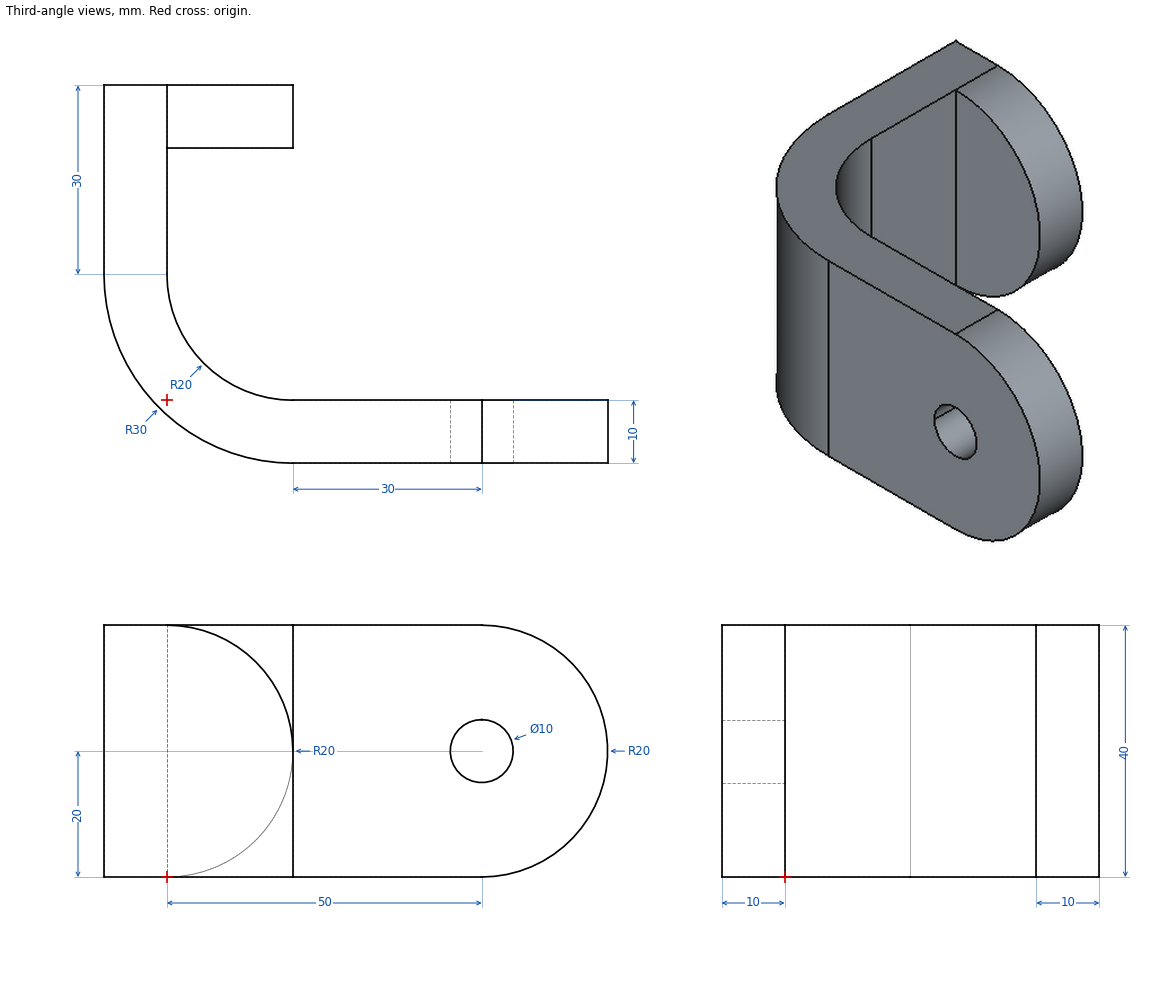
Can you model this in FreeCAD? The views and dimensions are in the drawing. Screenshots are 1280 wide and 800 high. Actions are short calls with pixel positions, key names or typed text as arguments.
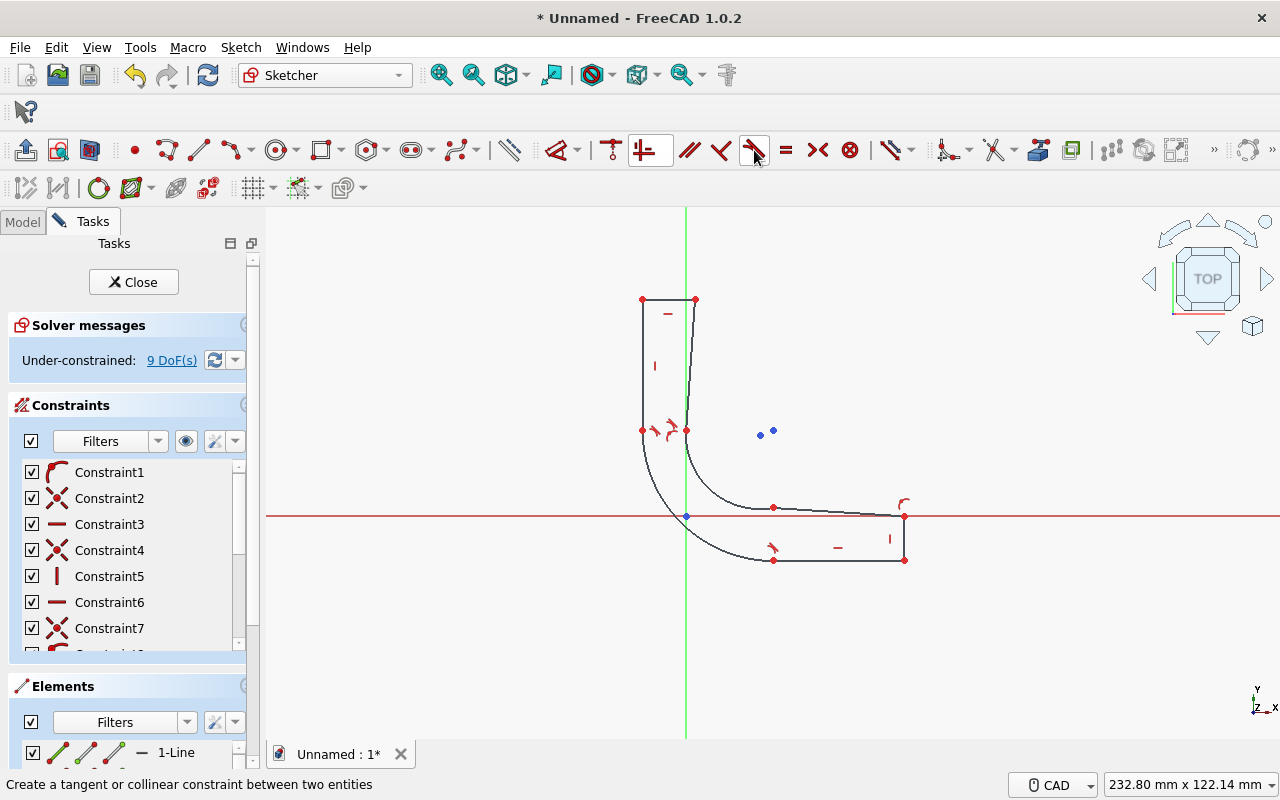
click(865, 514)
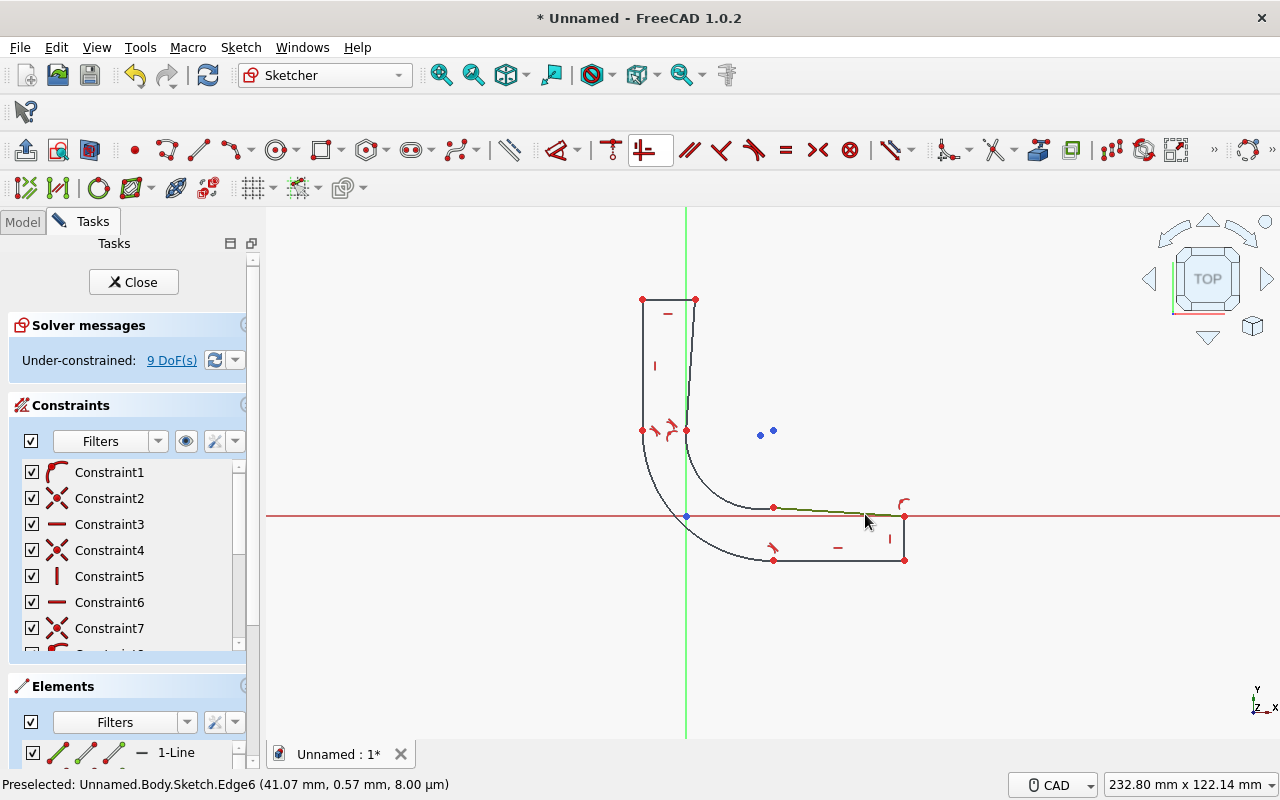
click(733, 504)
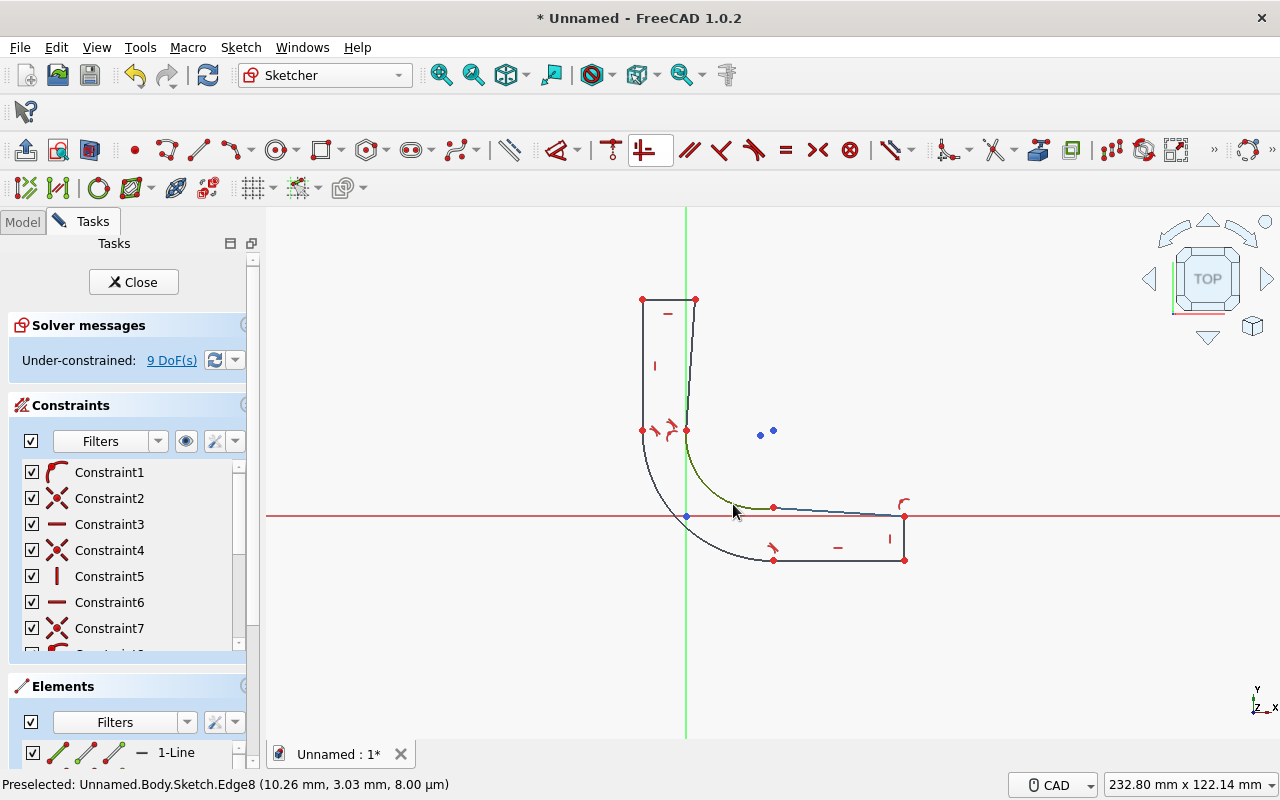
click(754, 150)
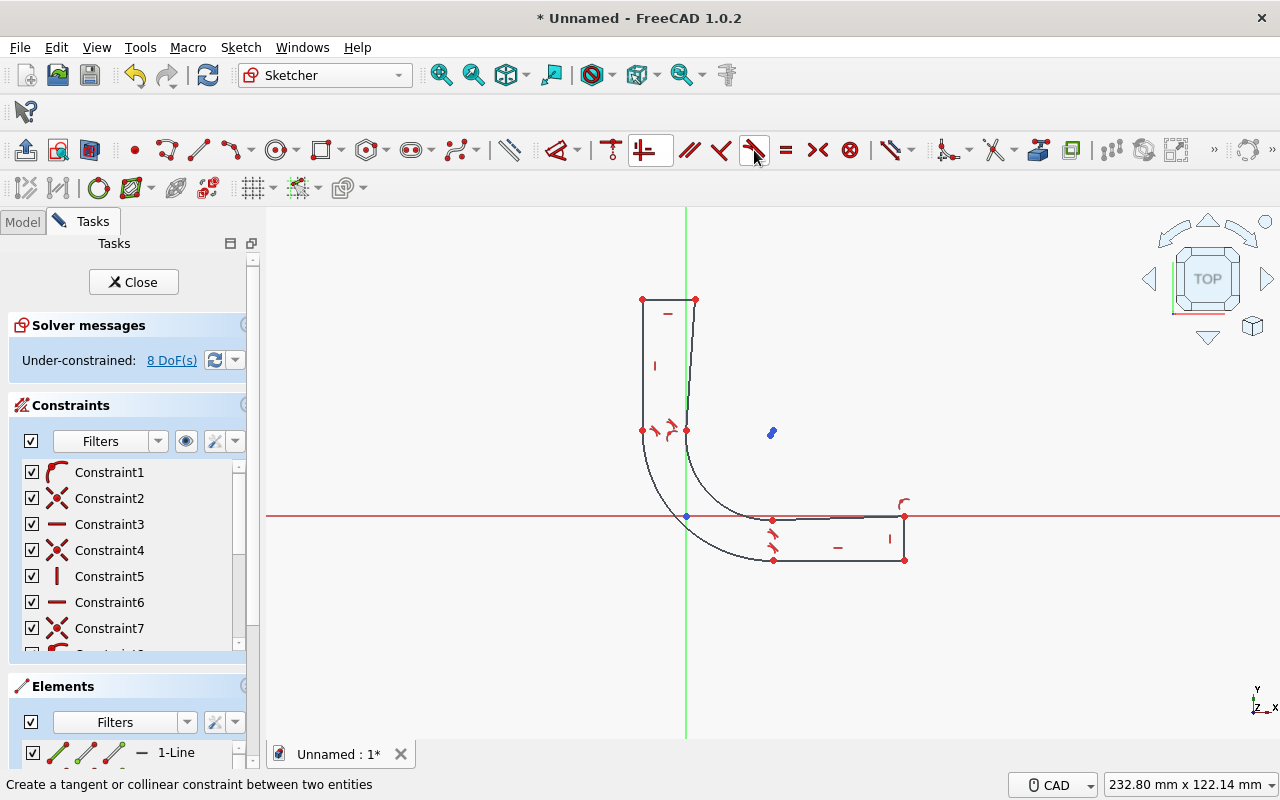
click(689, 391)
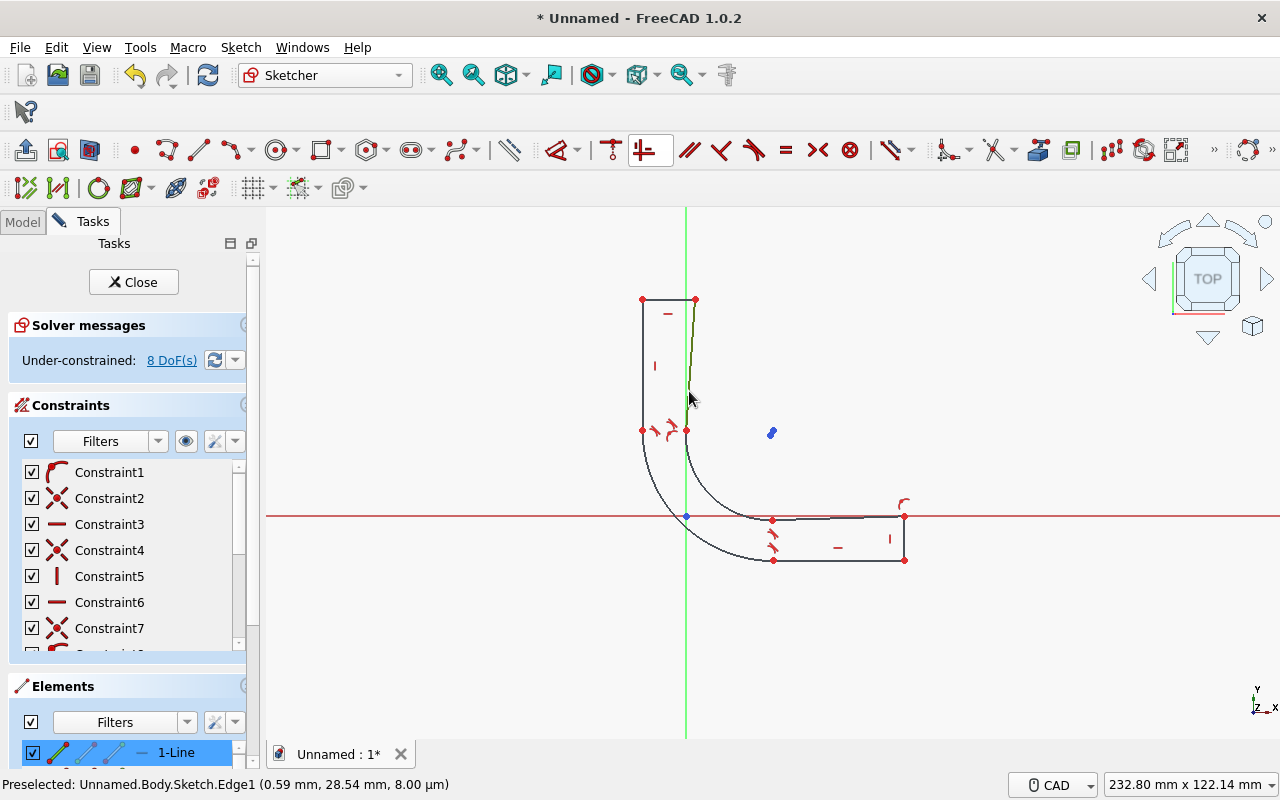
click(668, 150)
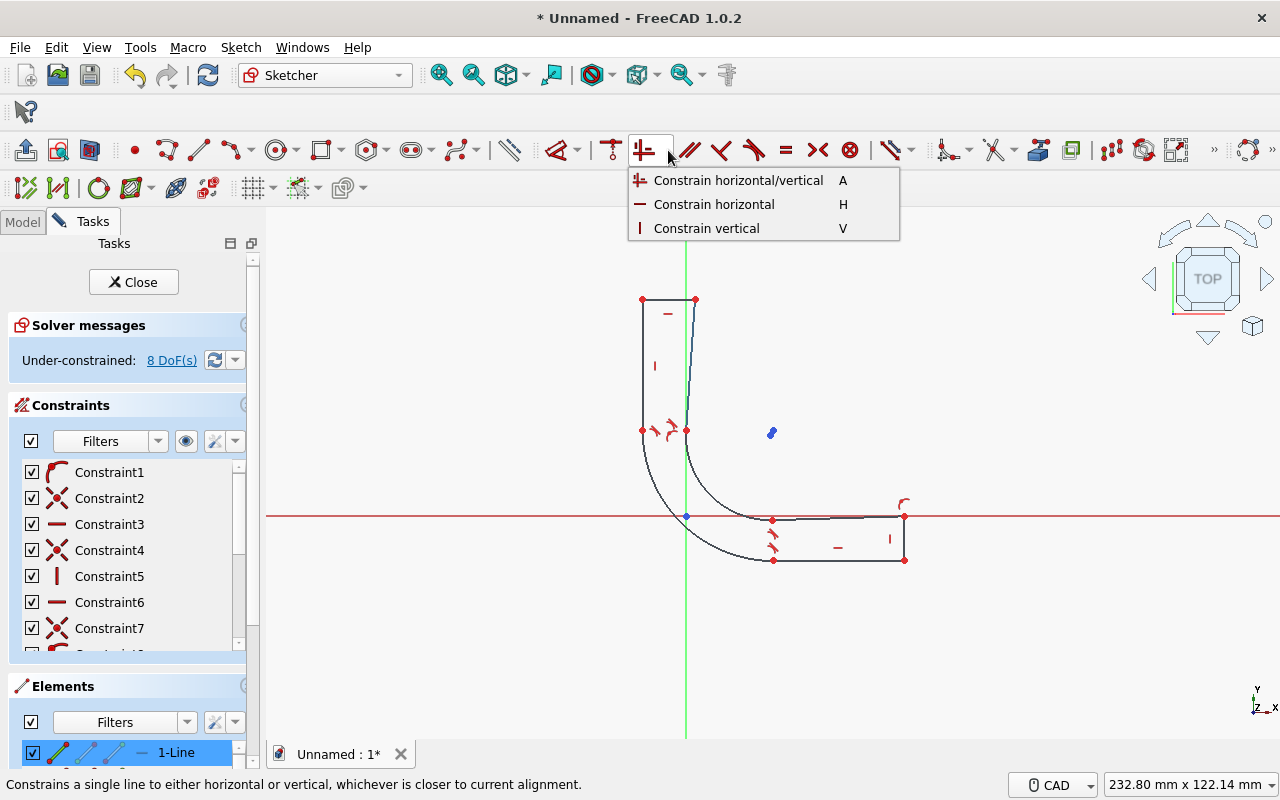
click(764, 228)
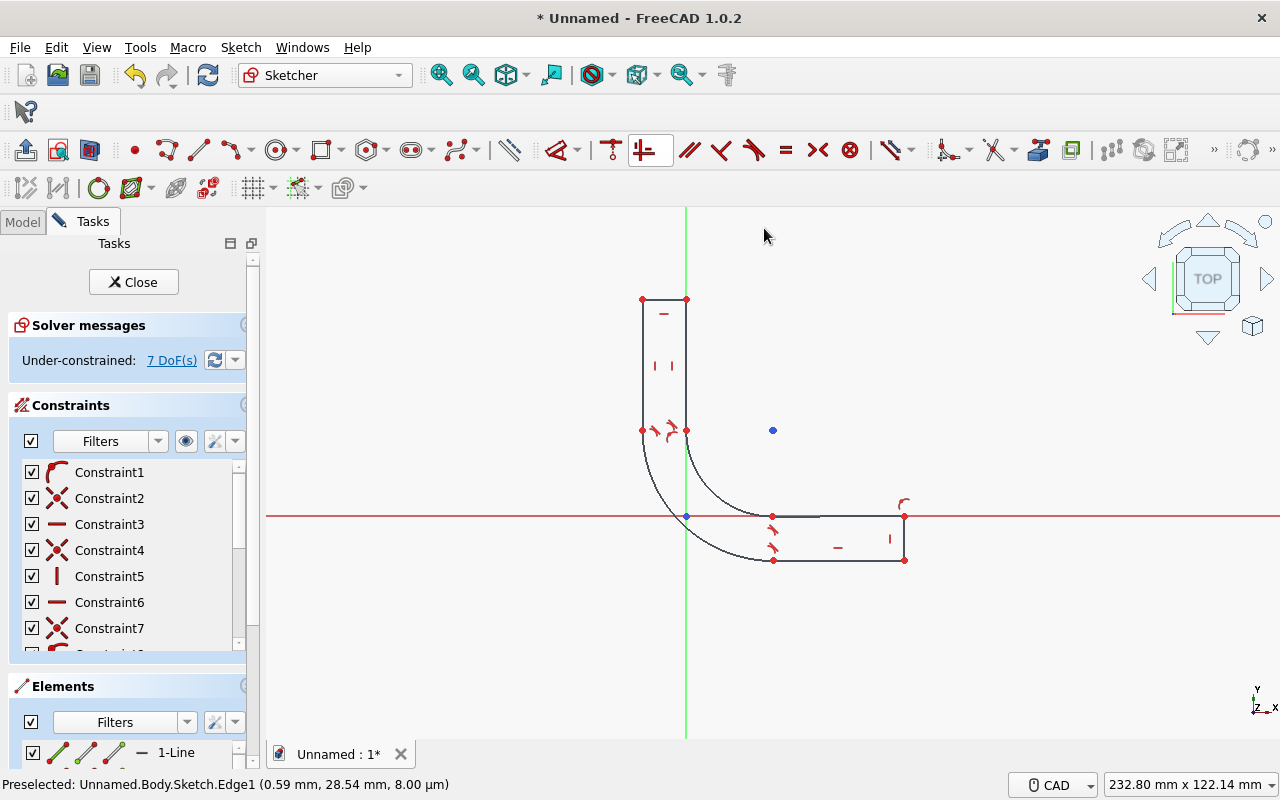
click(865, 516)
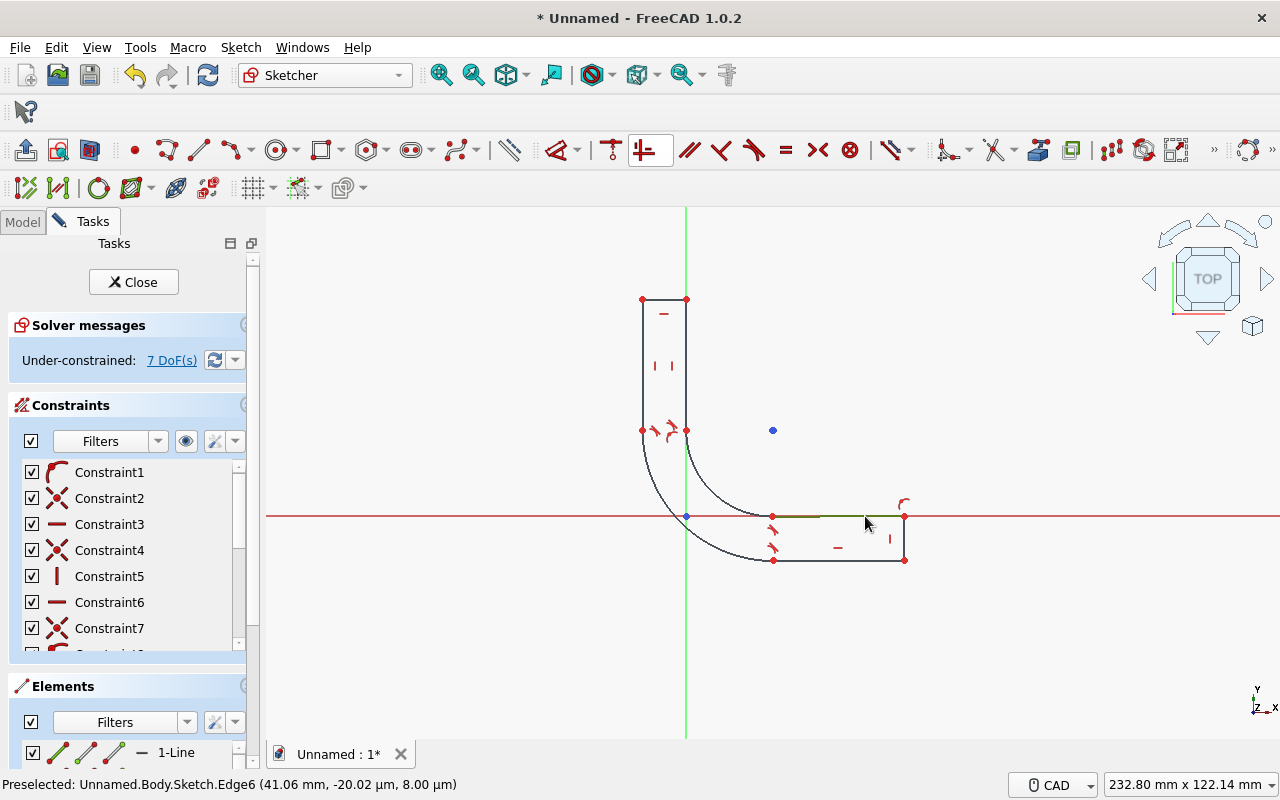
key(h)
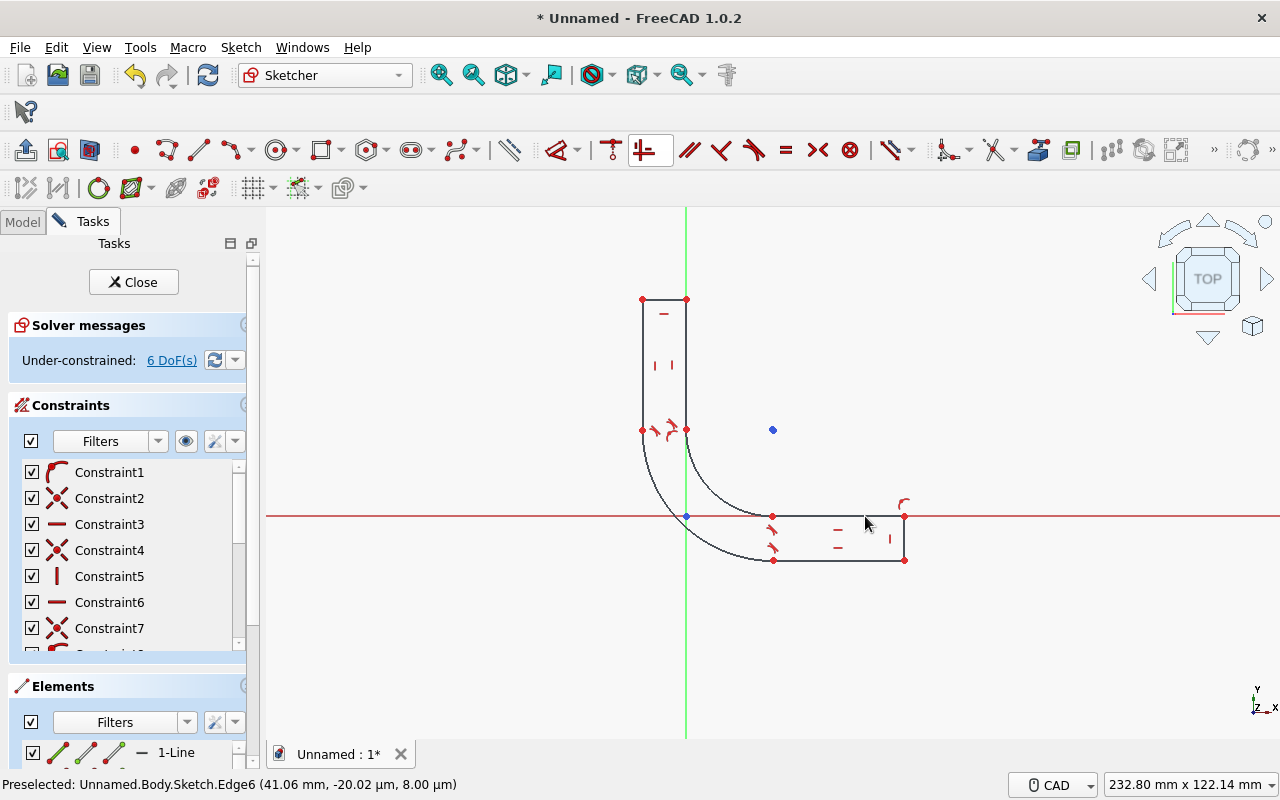
click(657, 489)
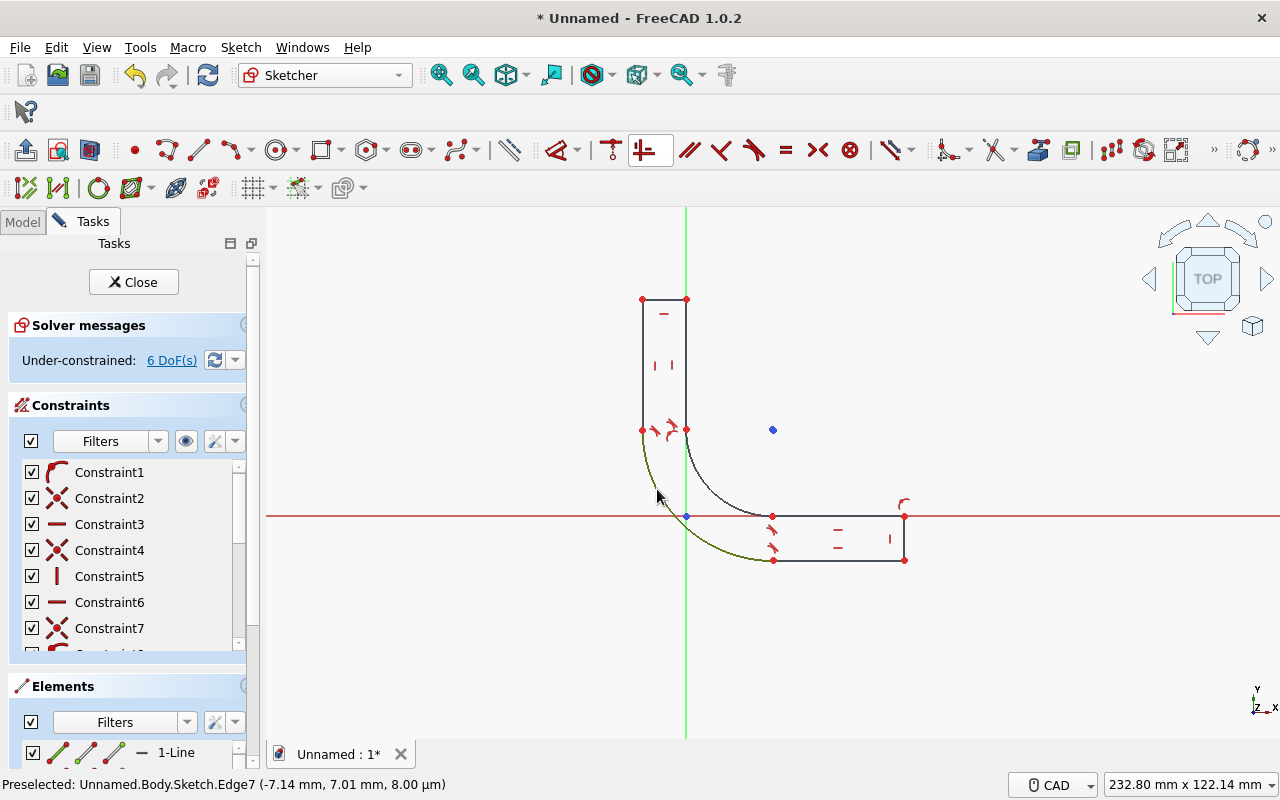
scroll(696, 469, up, 2)